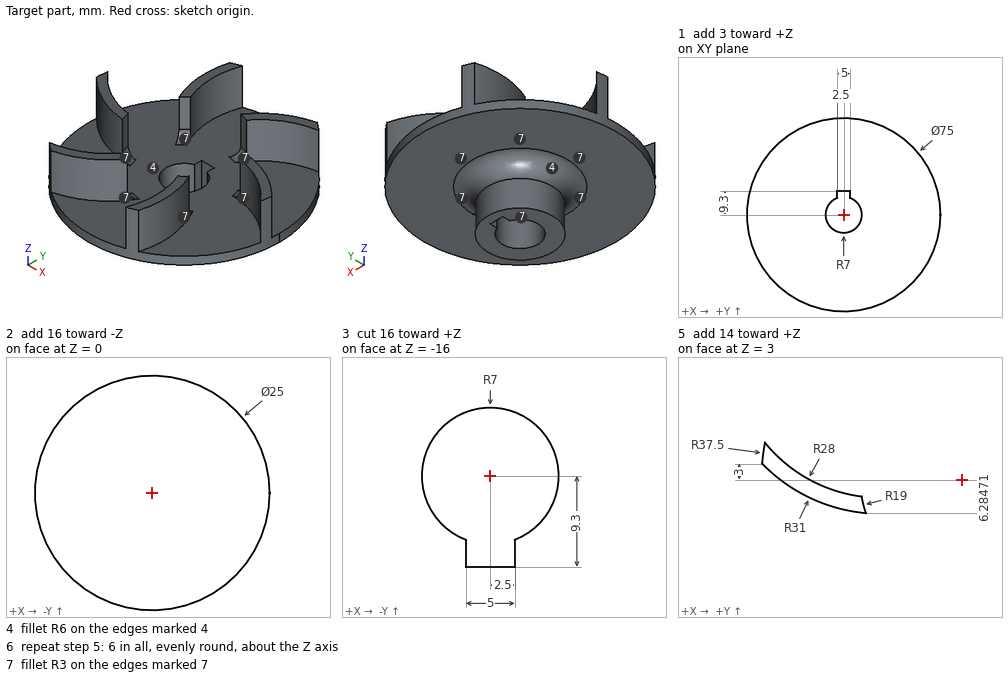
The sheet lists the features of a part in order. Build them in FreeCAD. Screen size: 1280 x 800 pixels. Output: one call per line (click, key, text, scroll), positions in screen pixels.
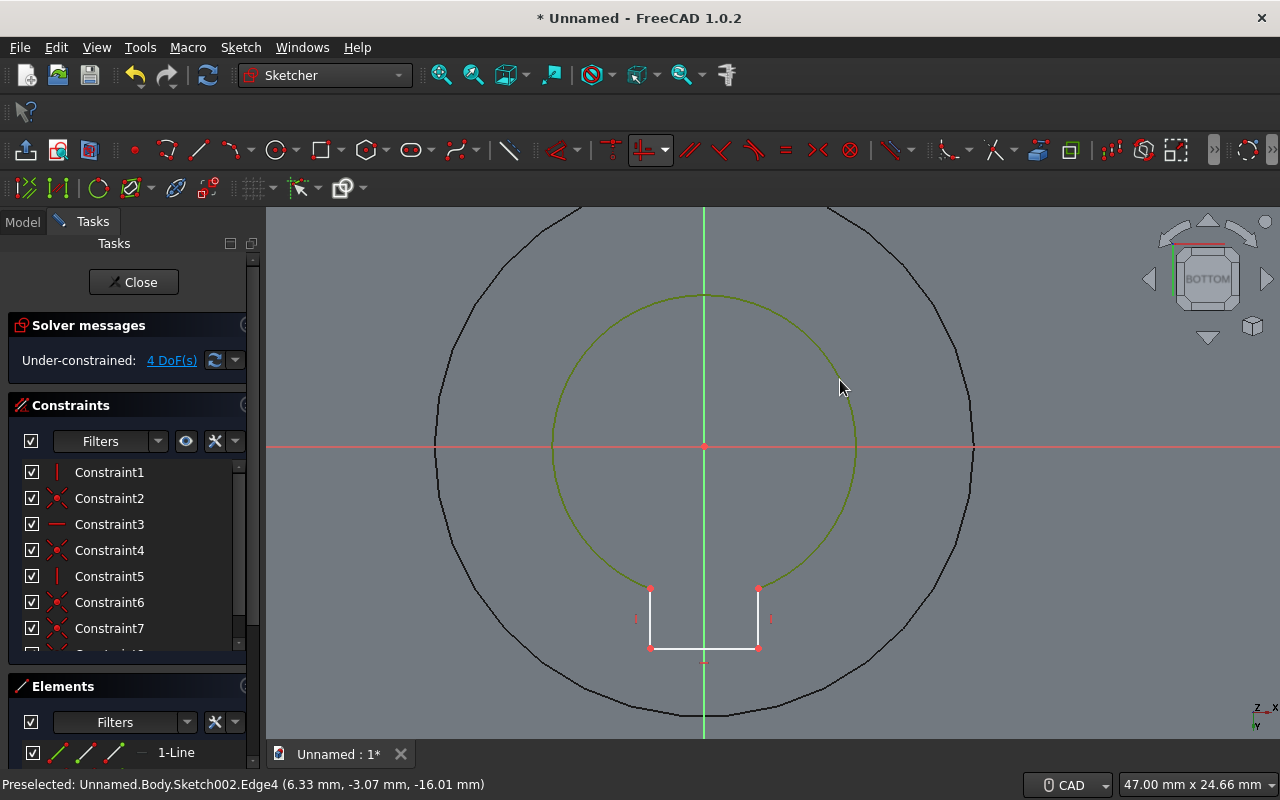
key(k)
key(r)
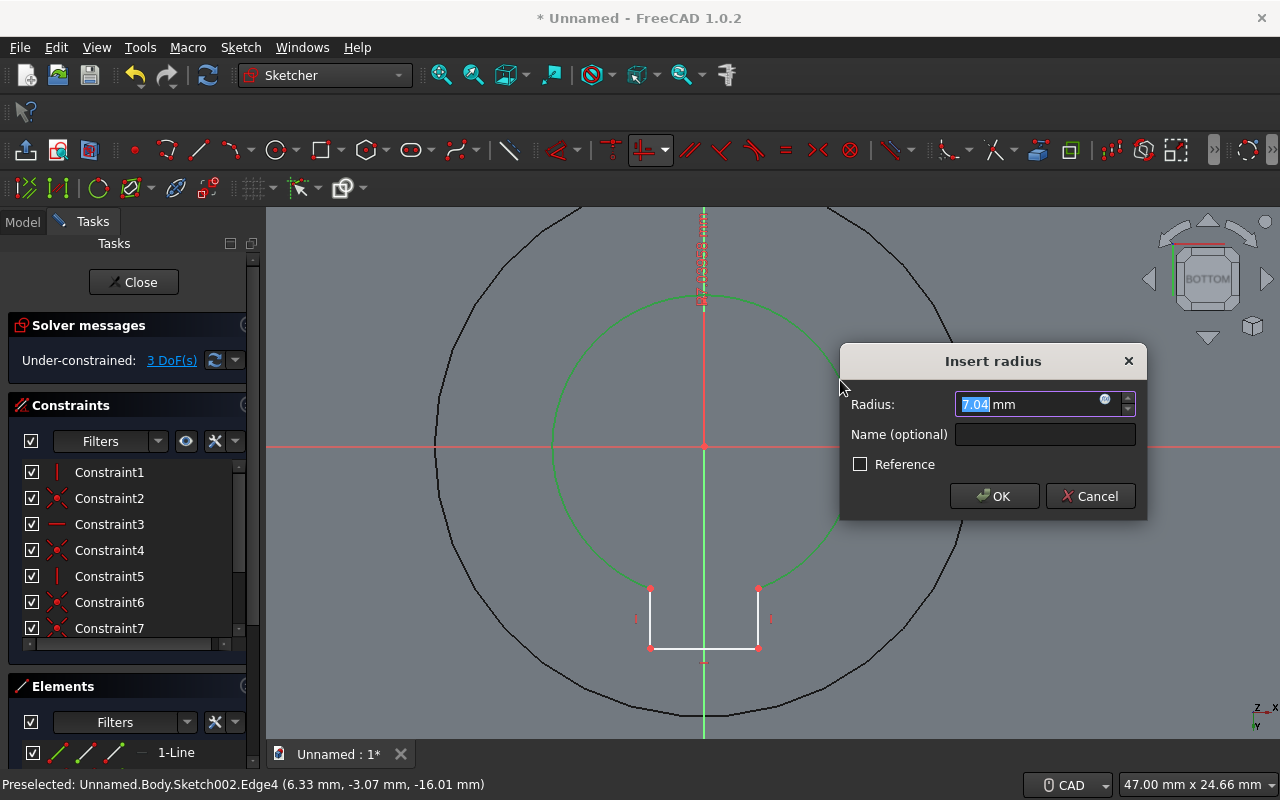
text(7)
key(Return)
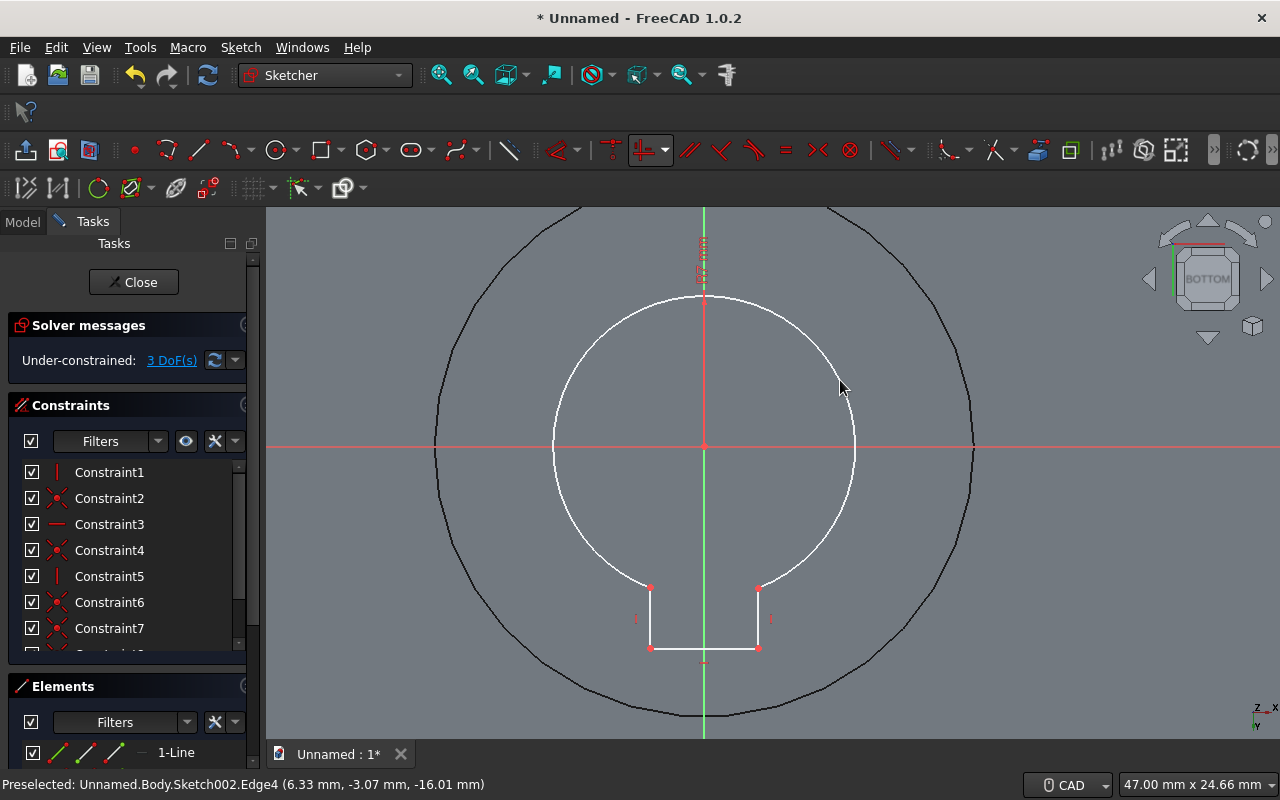
click(726, 649)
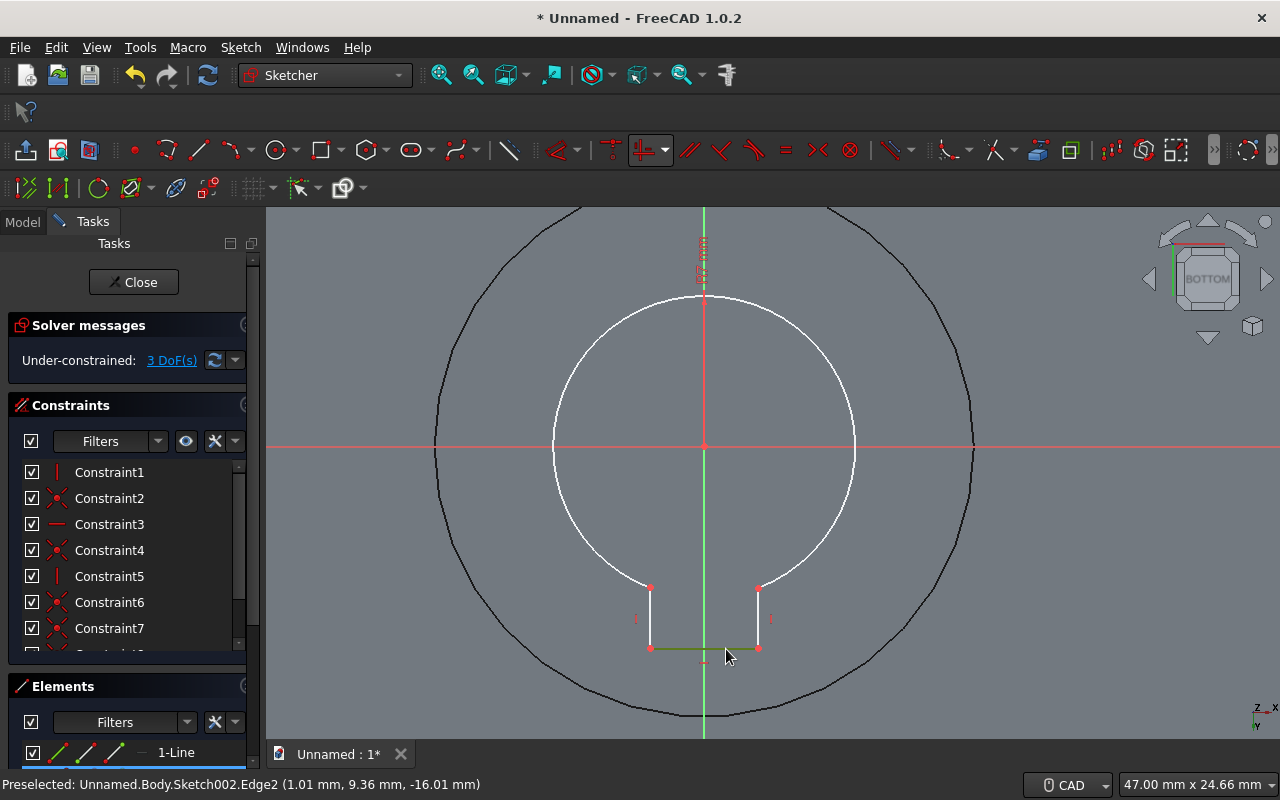
key(l)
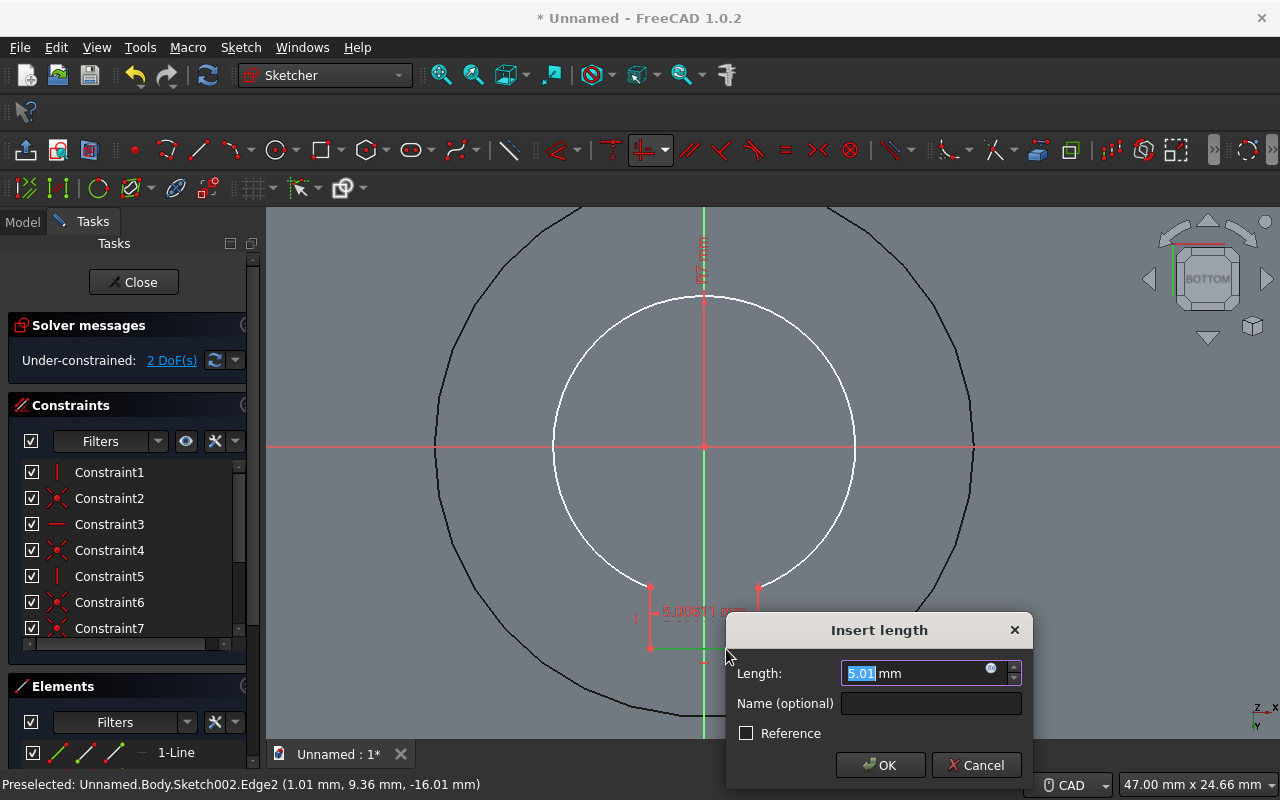
text(5)
key(Return)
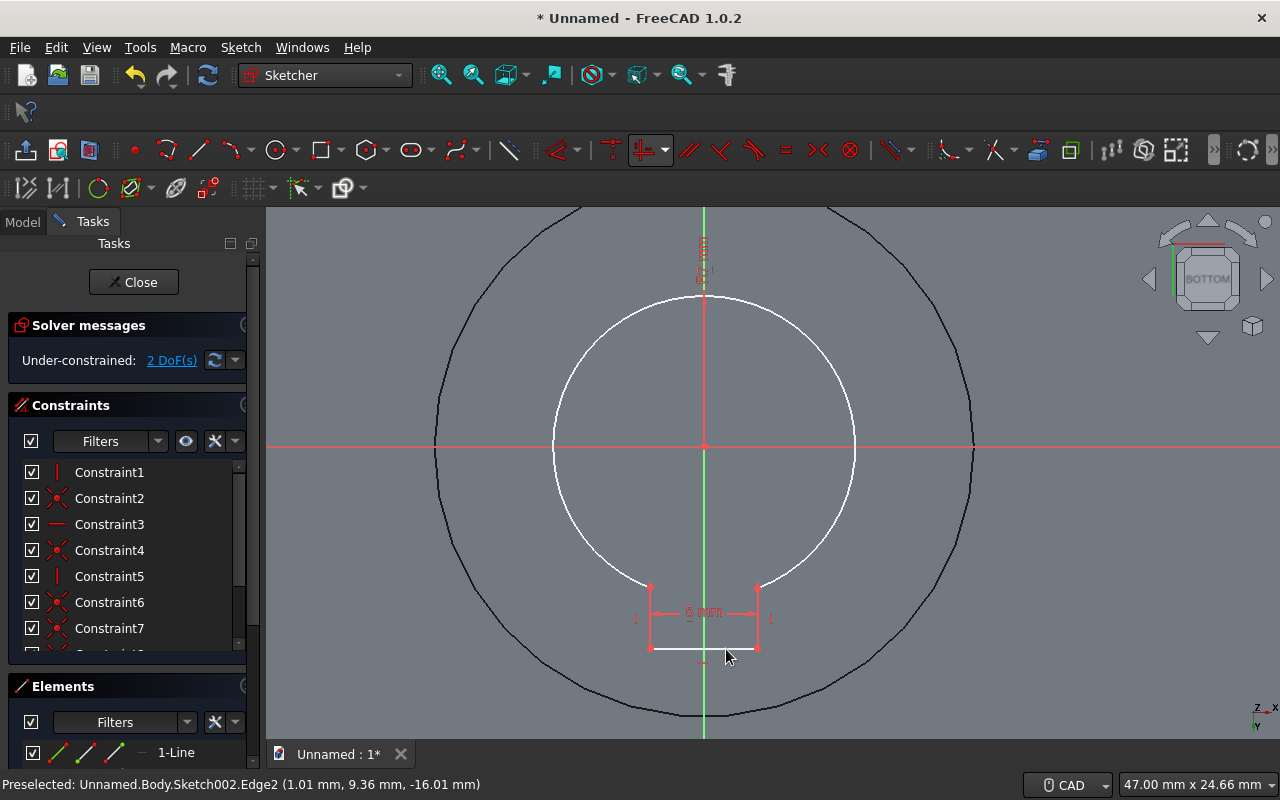
click(758, 588)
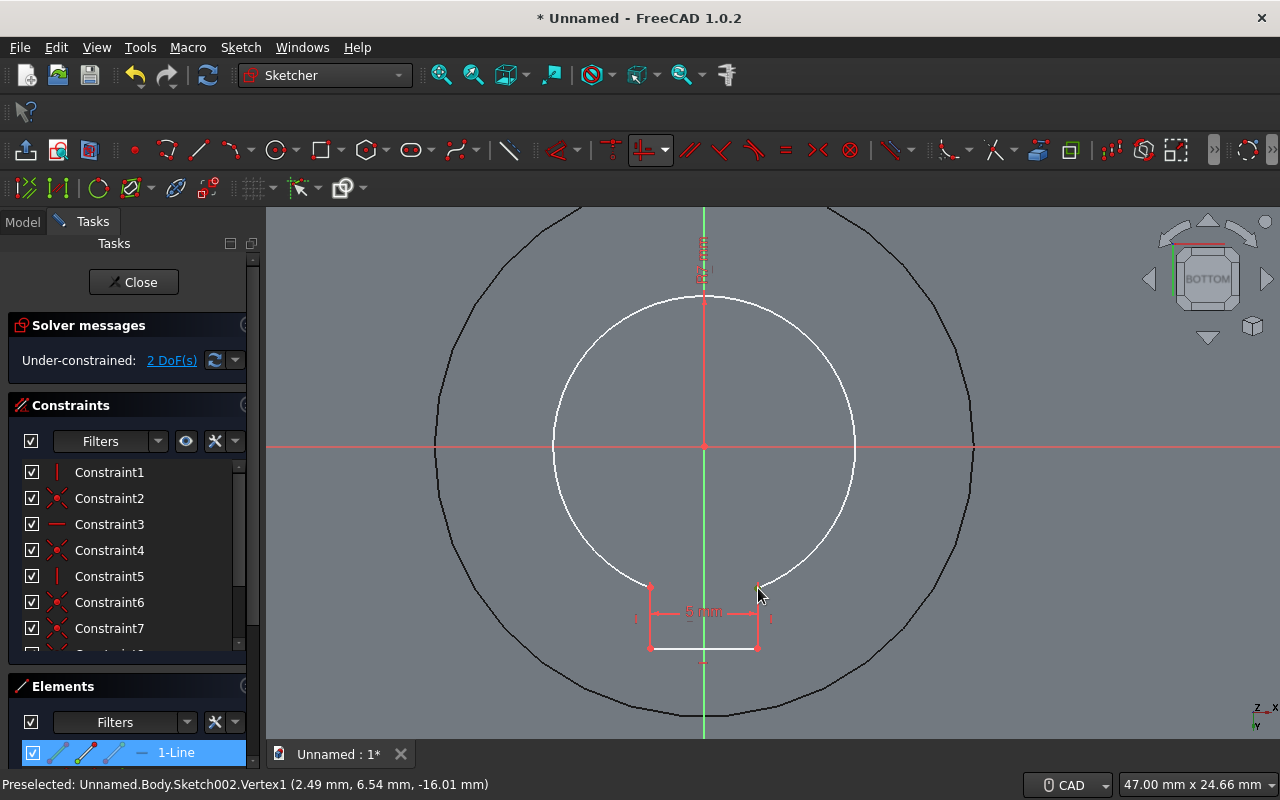
key(l)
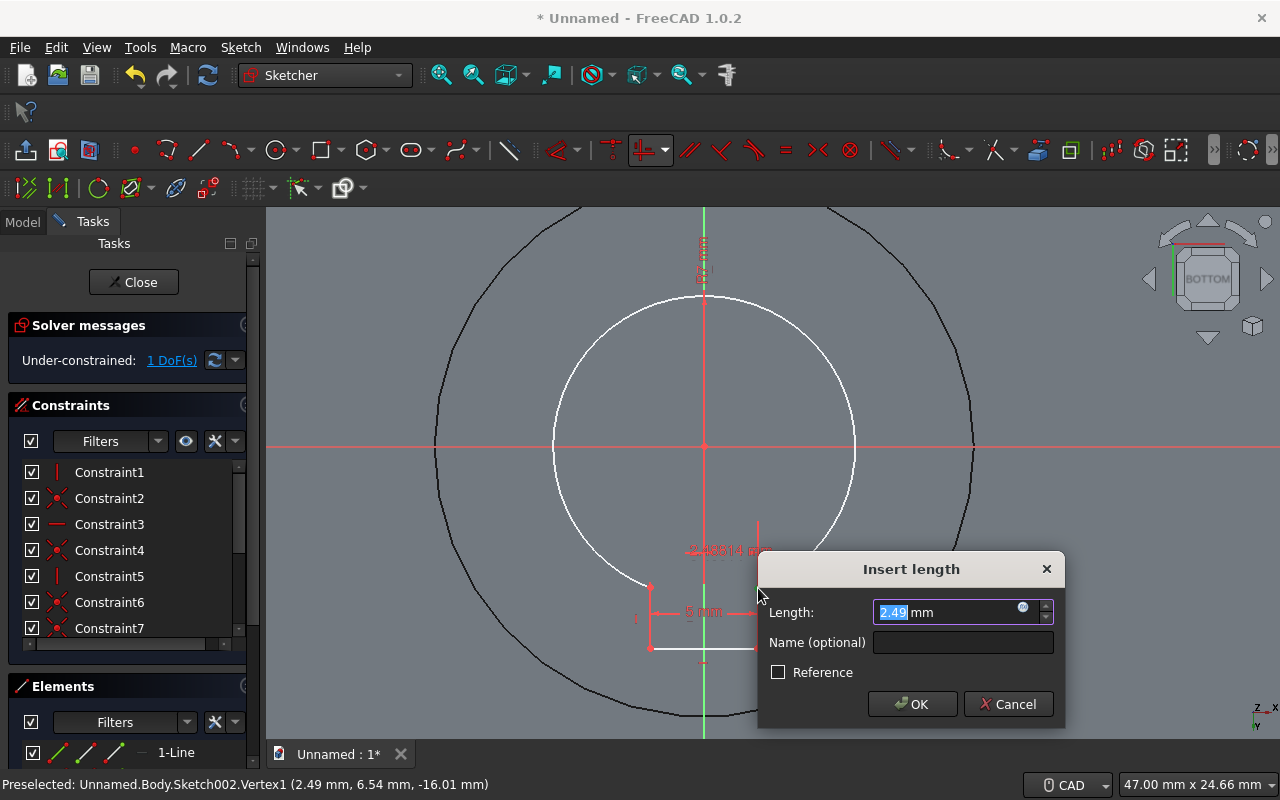
text(2.5)
key(Return)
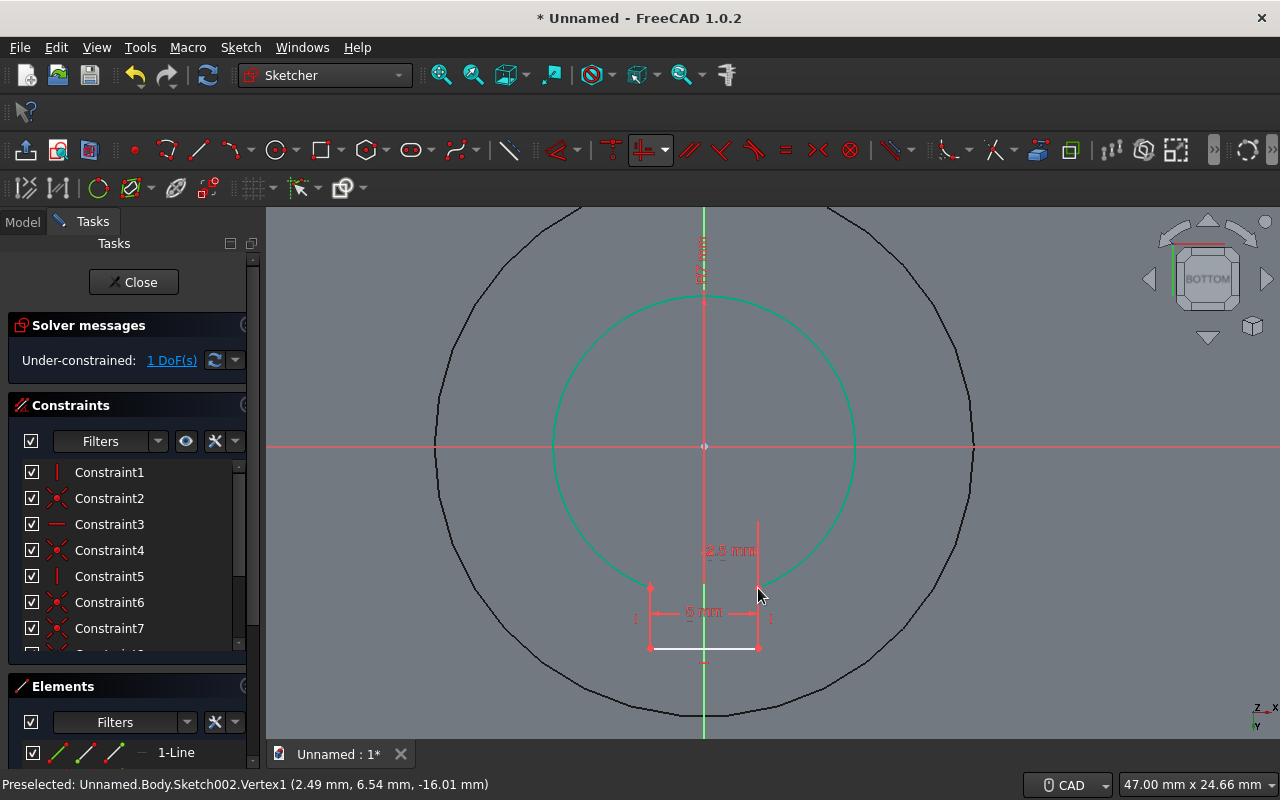
click(758, 649)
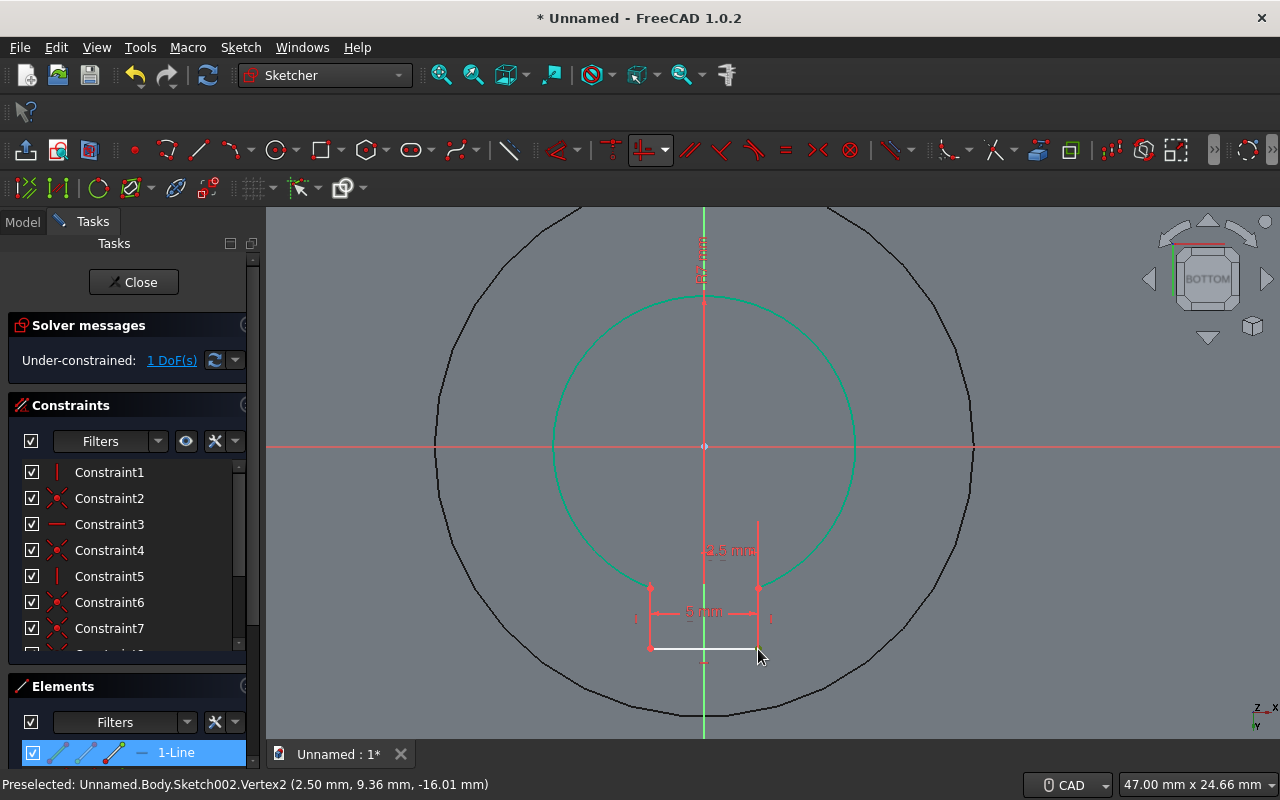
click(580, 150)